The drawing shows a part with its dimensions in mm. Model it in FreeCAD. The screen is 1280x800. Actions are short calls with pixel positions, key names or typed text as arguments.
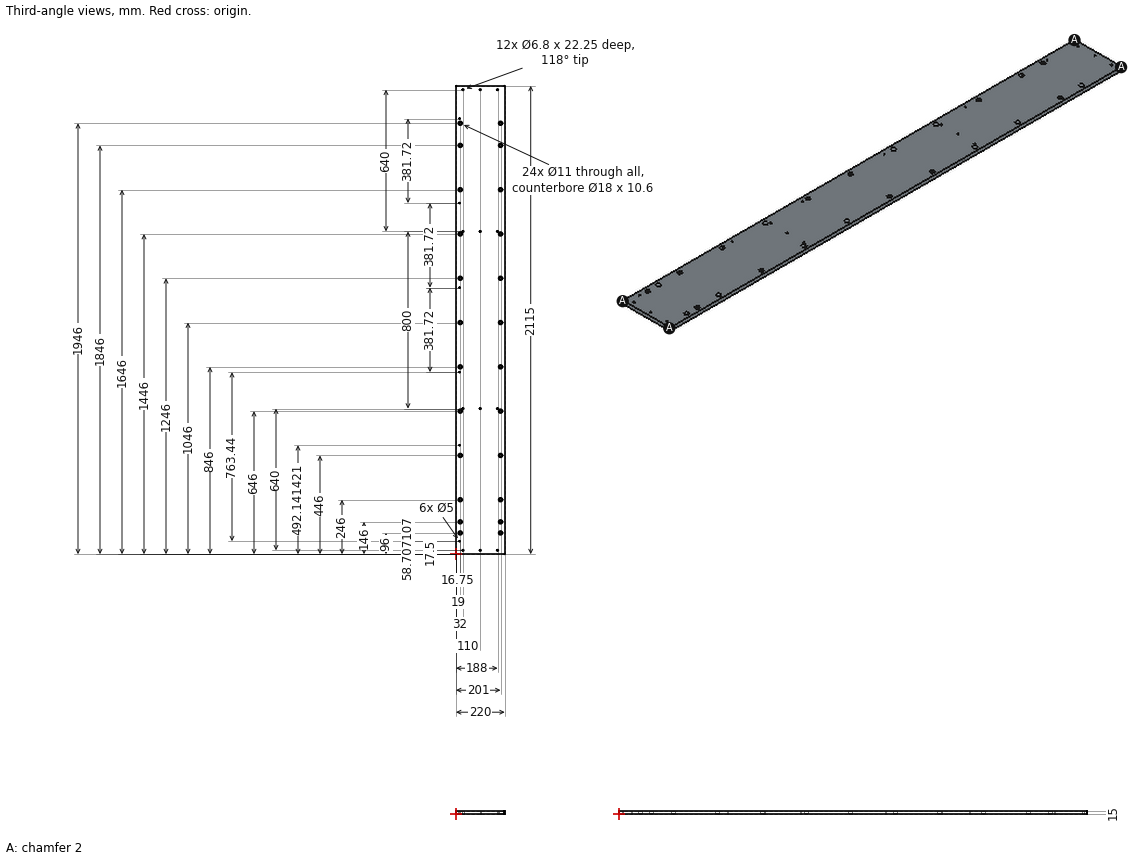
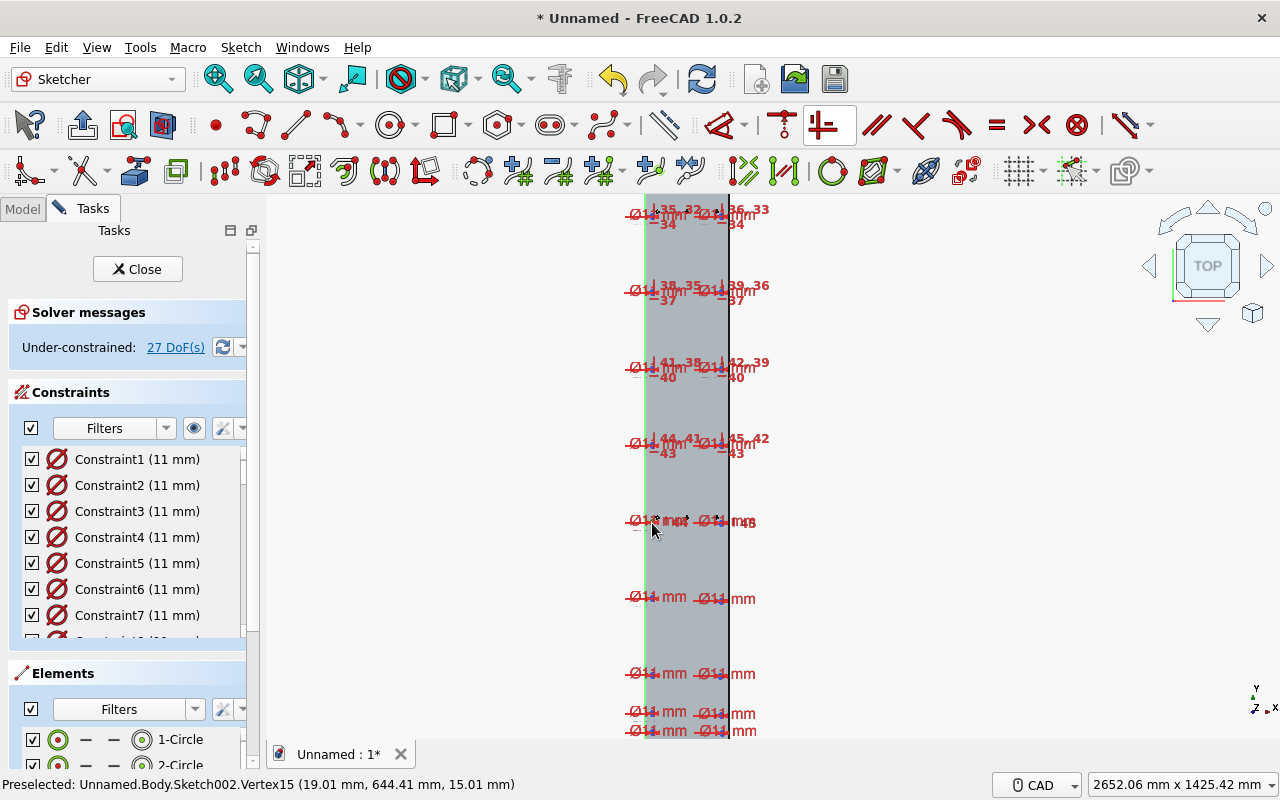
click(721, 523)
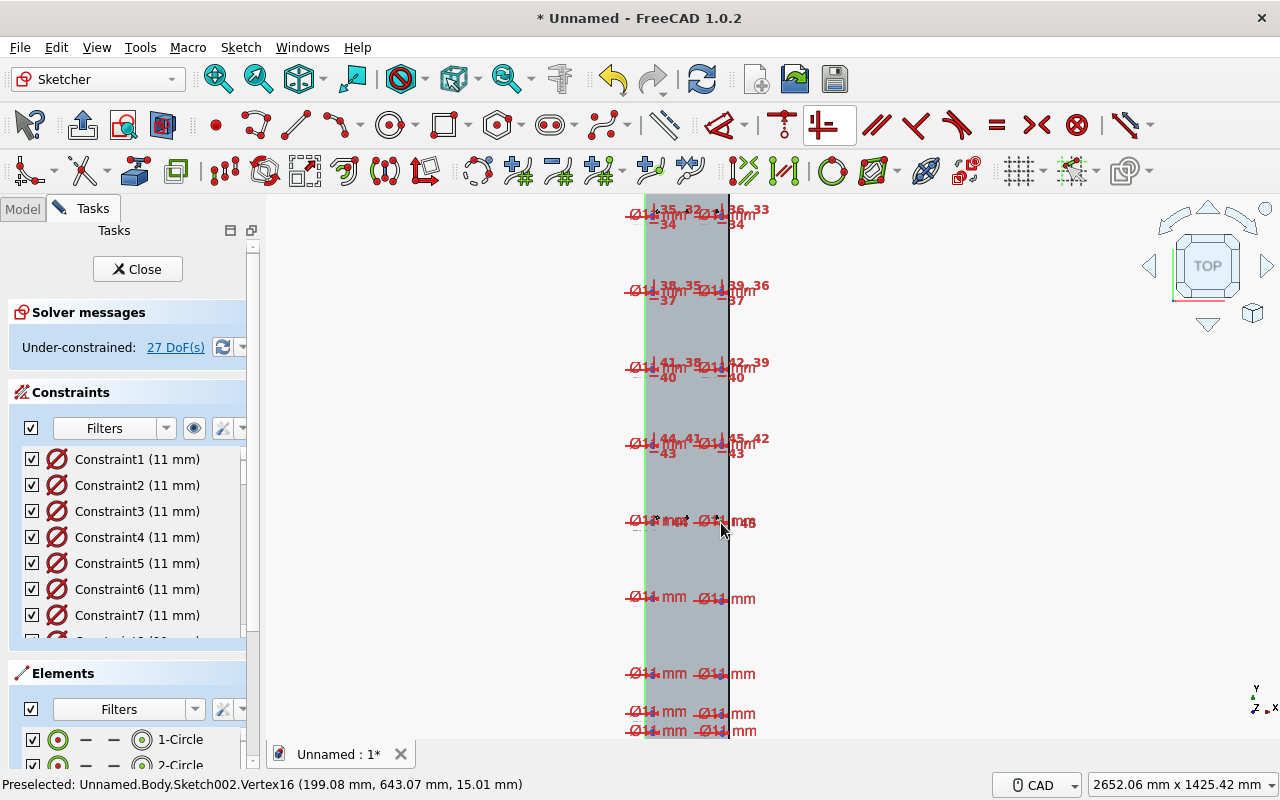
key(h)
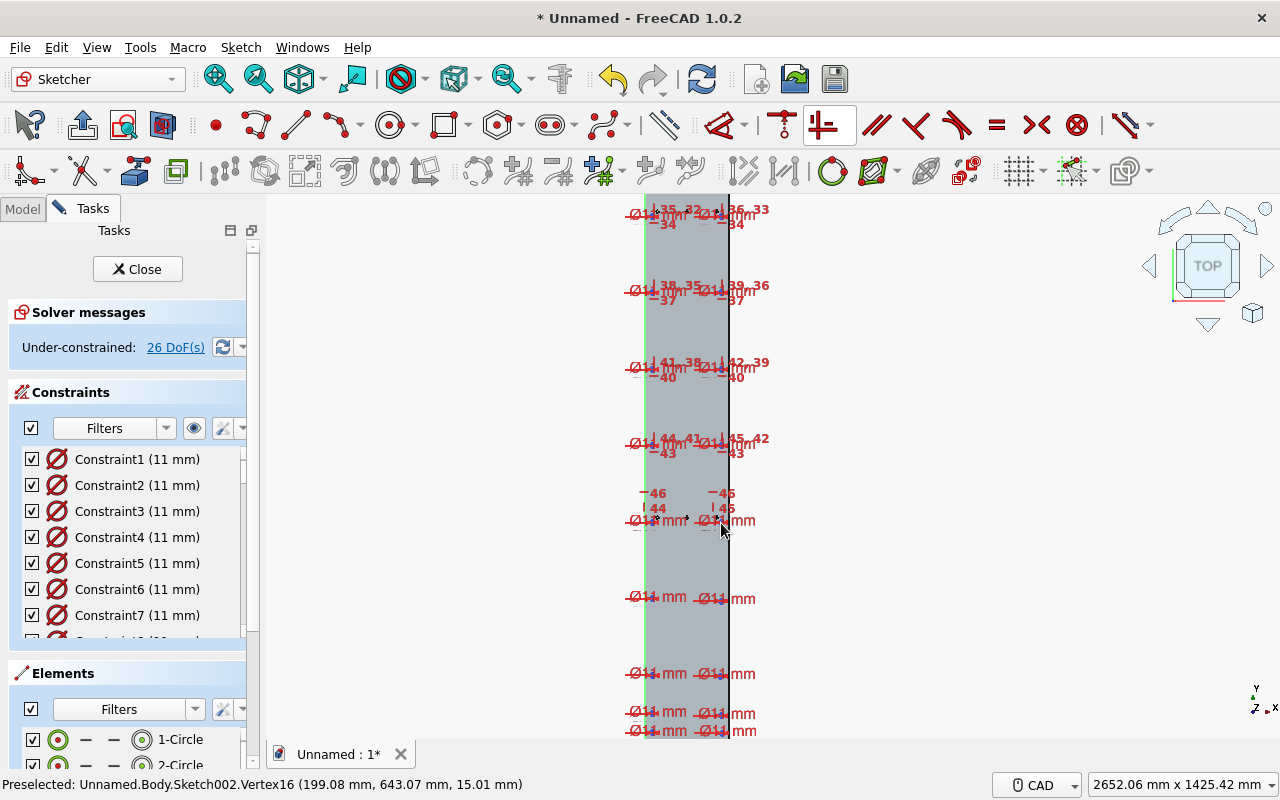
click(652, 523)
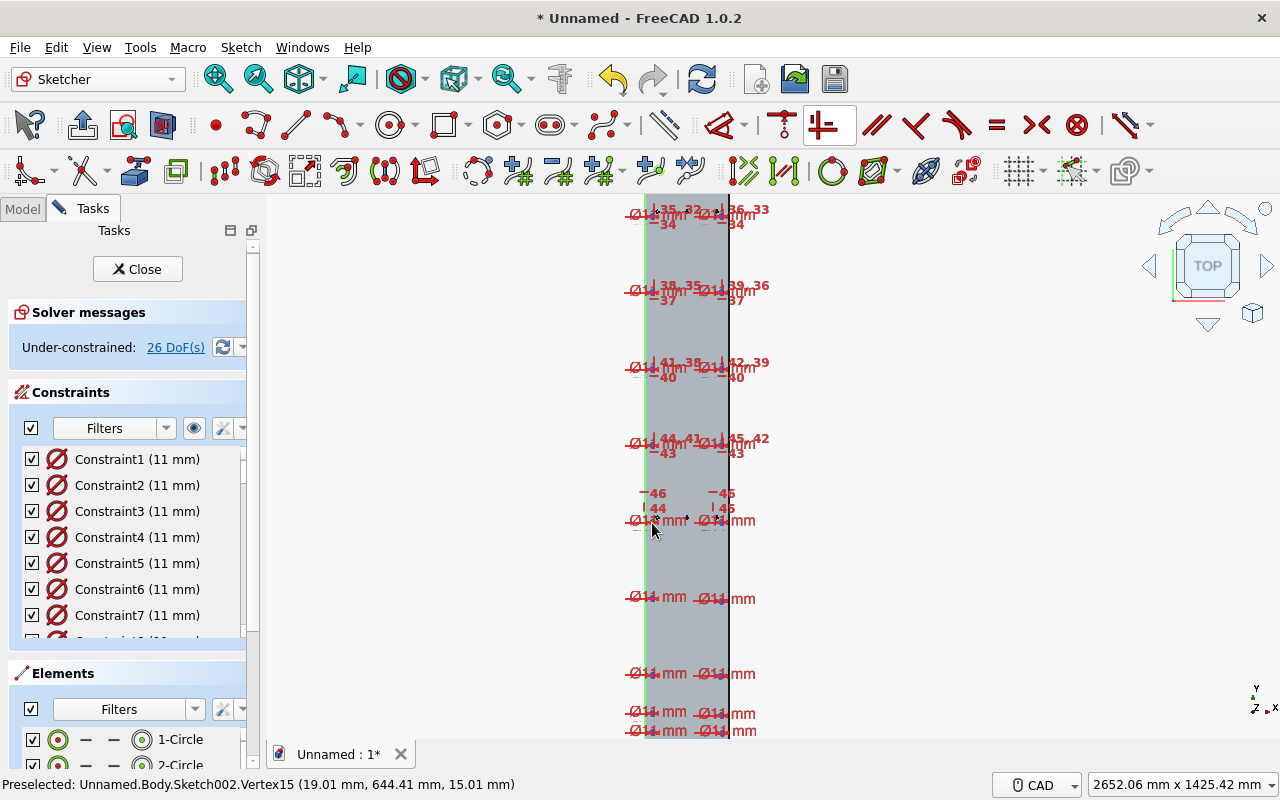
click(652, 599)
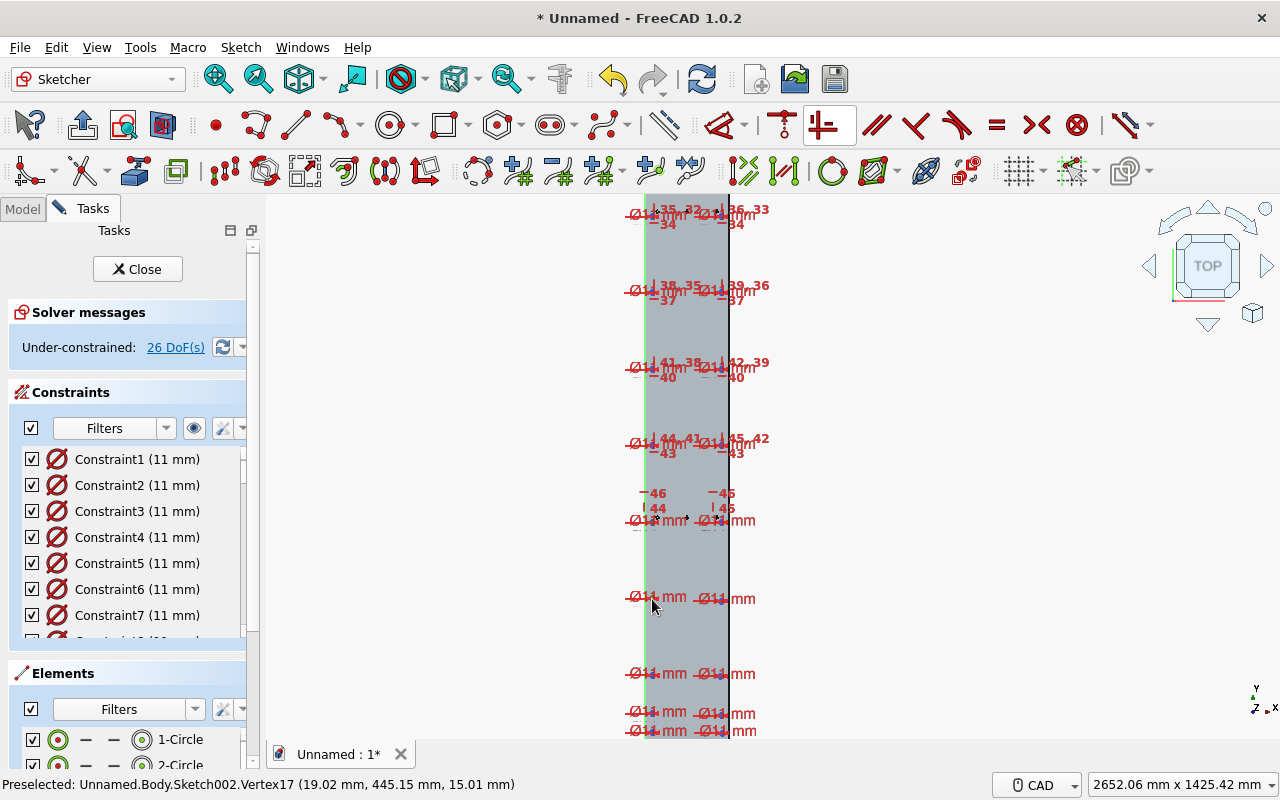
click(850, 126)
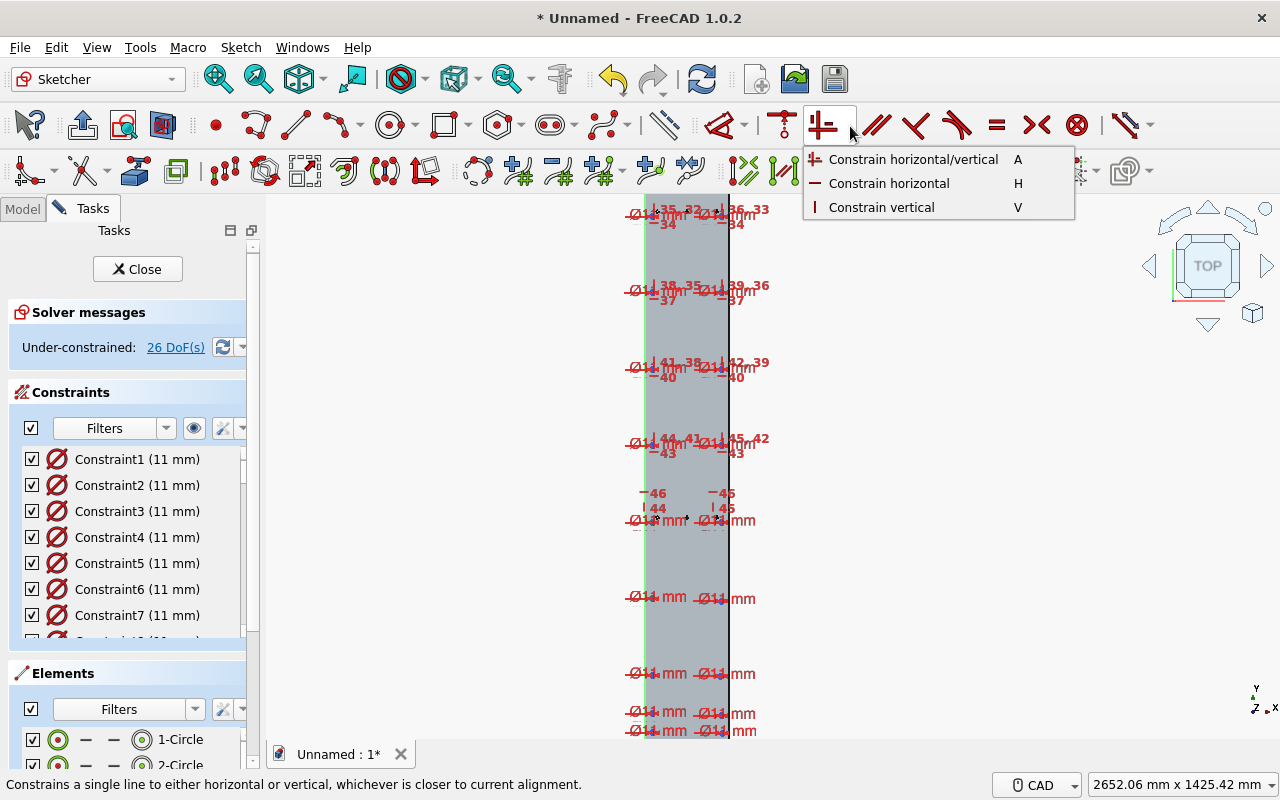
click(939, 207)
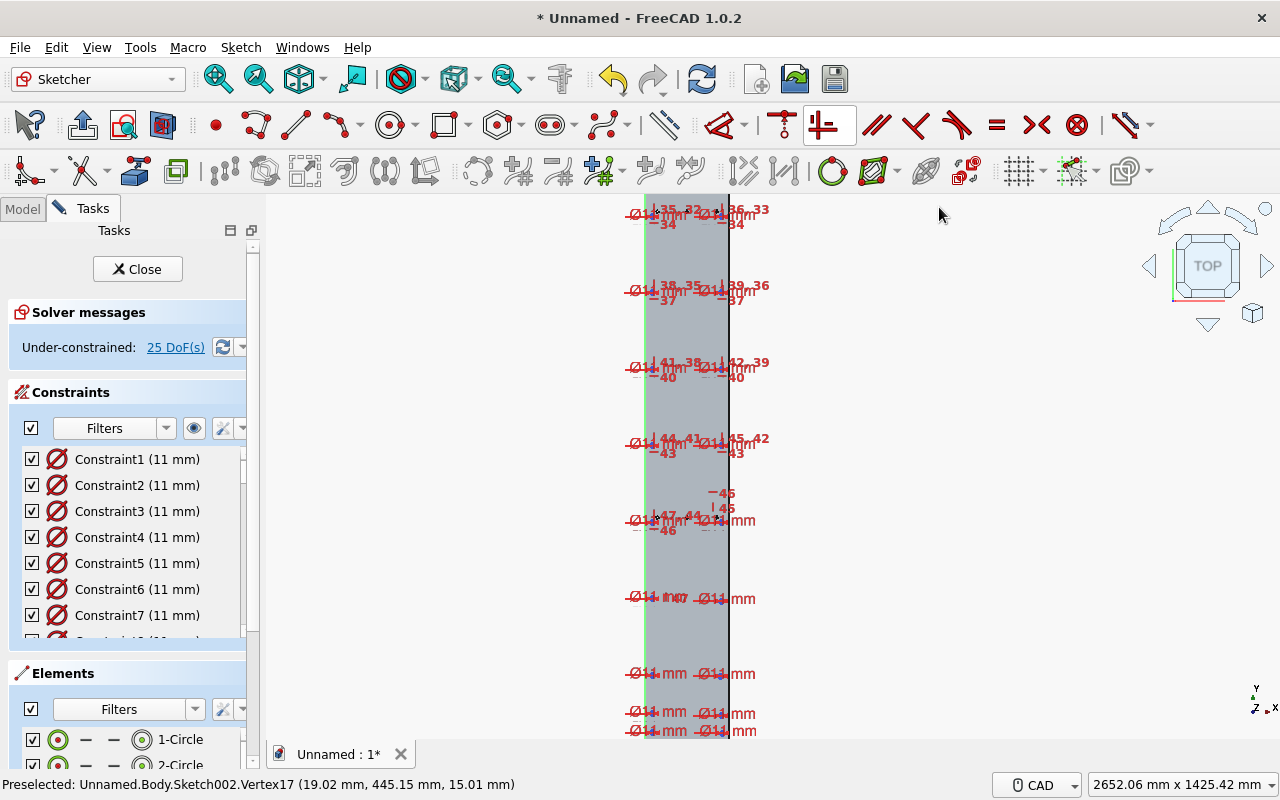
click(721, 523)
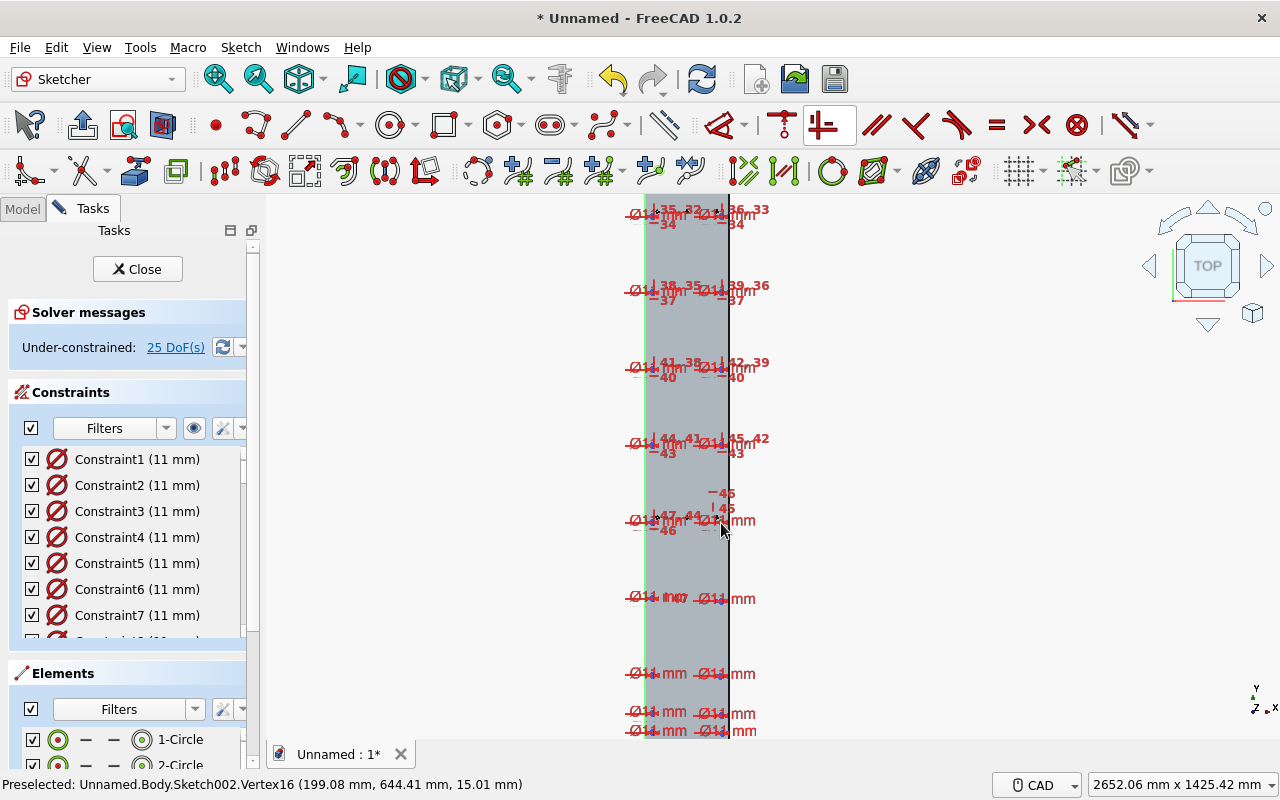
click(721, 601)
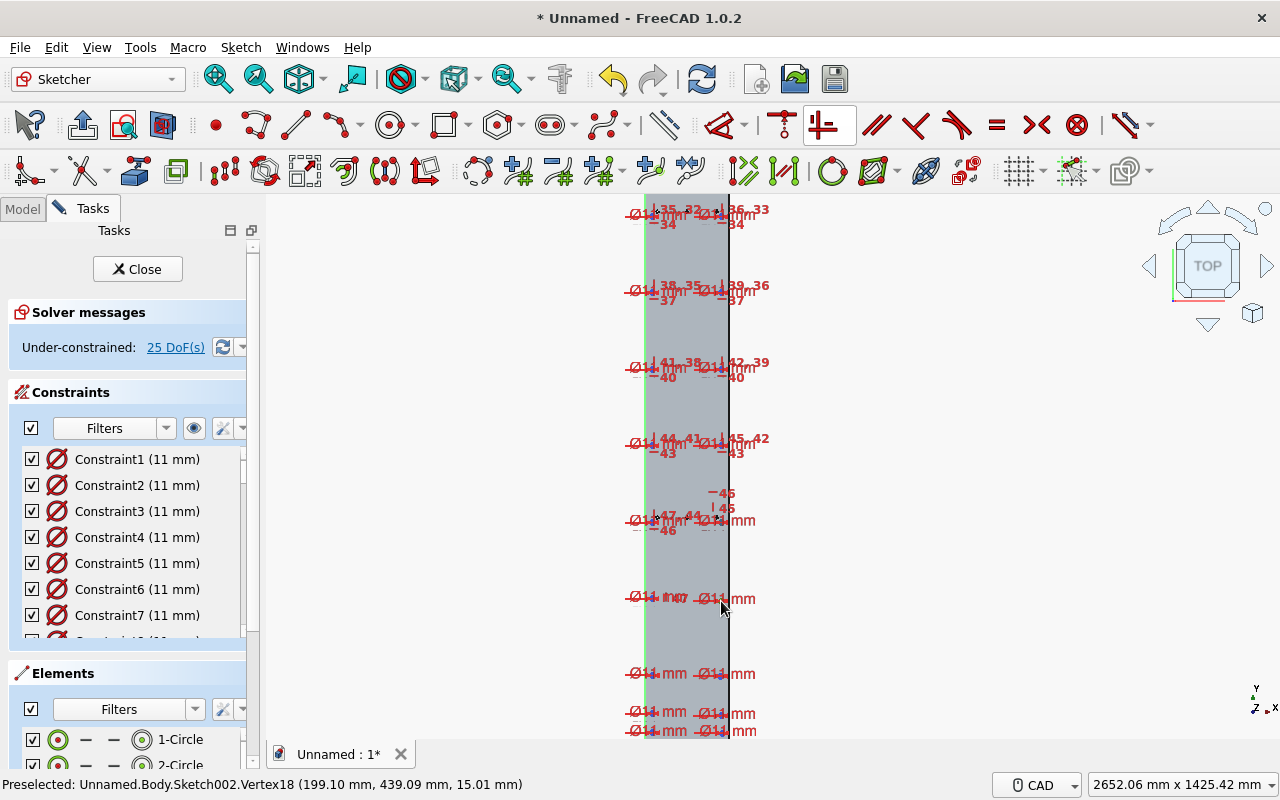
click(850, 126)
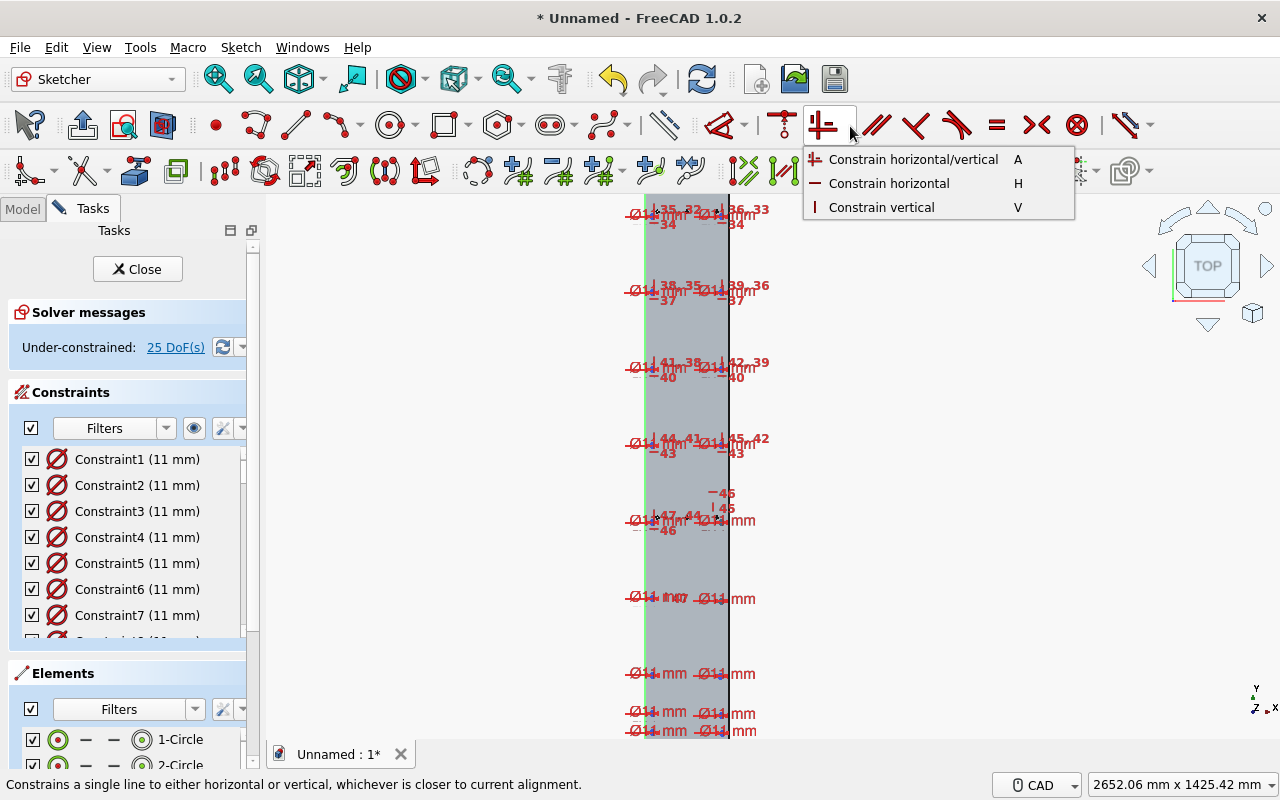
click(939, 207)